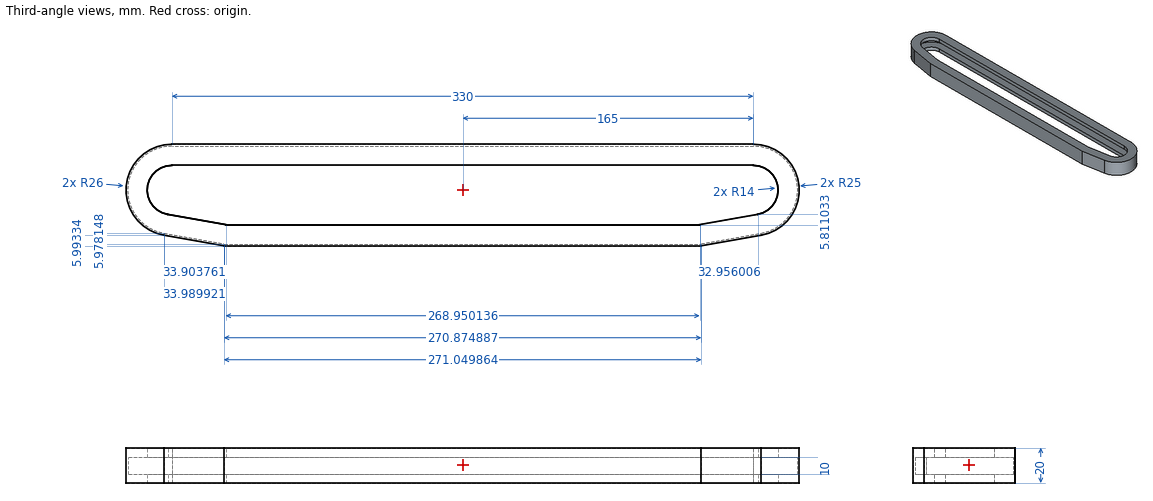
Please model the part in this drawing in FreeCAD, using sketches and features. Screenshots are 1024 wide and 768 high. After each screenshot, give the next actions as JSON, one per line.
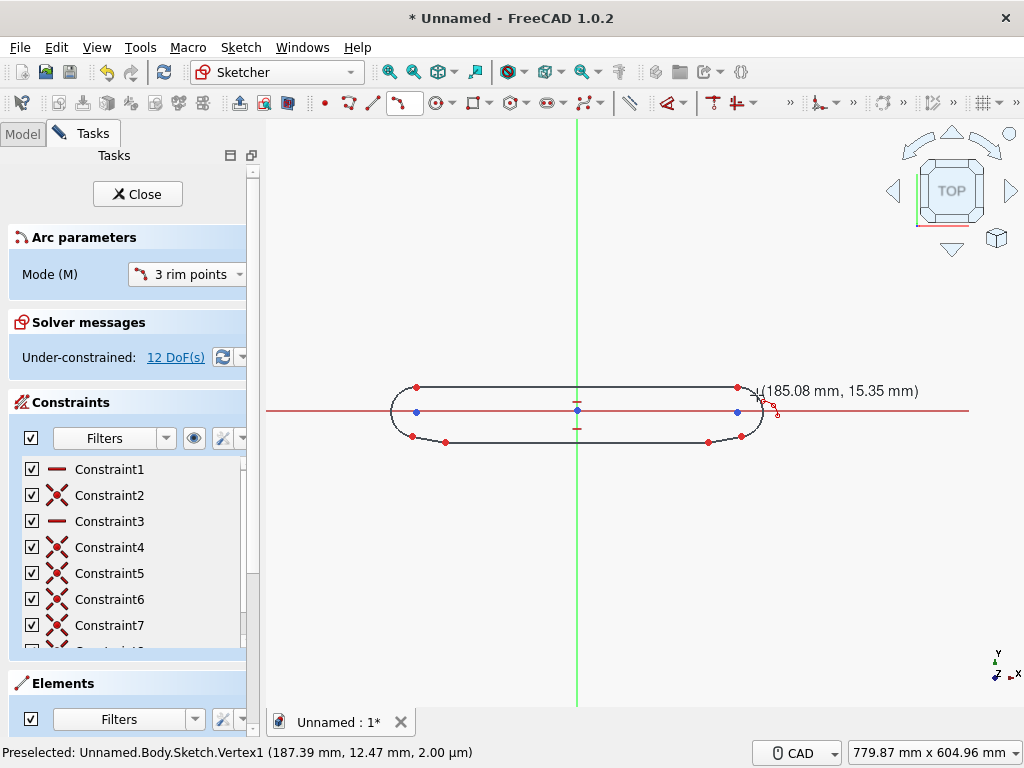
{"action": "left_click", "coordinate": [374, 104]}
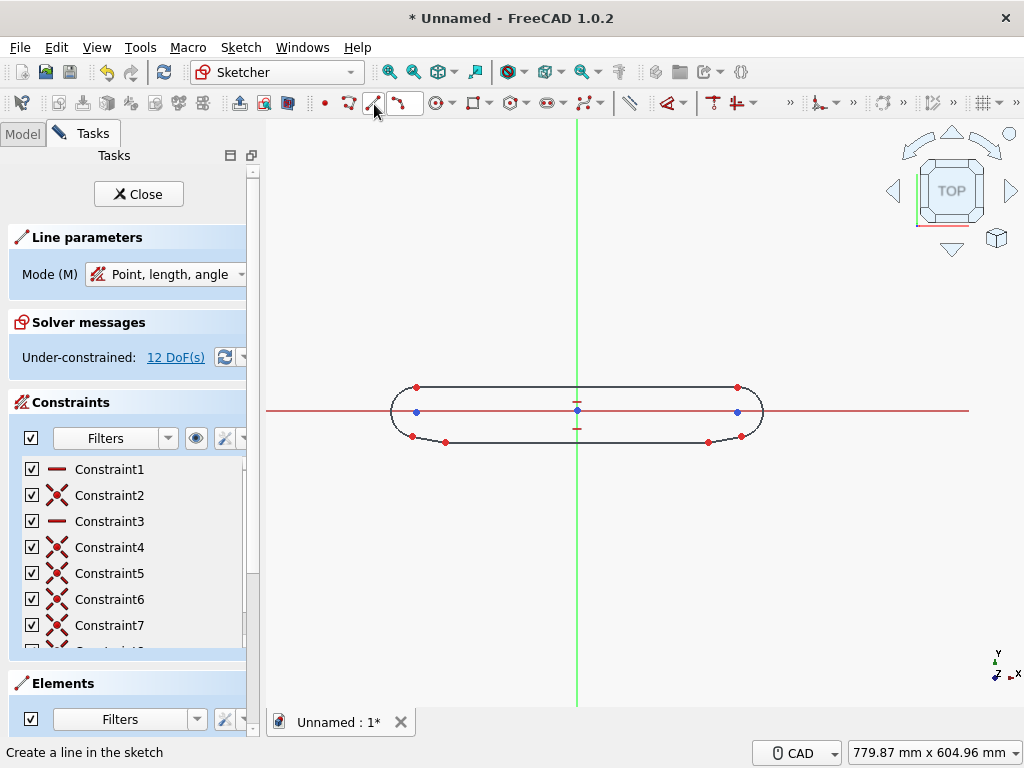
{"action": "scroll", "coordinate": [417, 397], "scroll_direction": "up", "scroll_amount": 2}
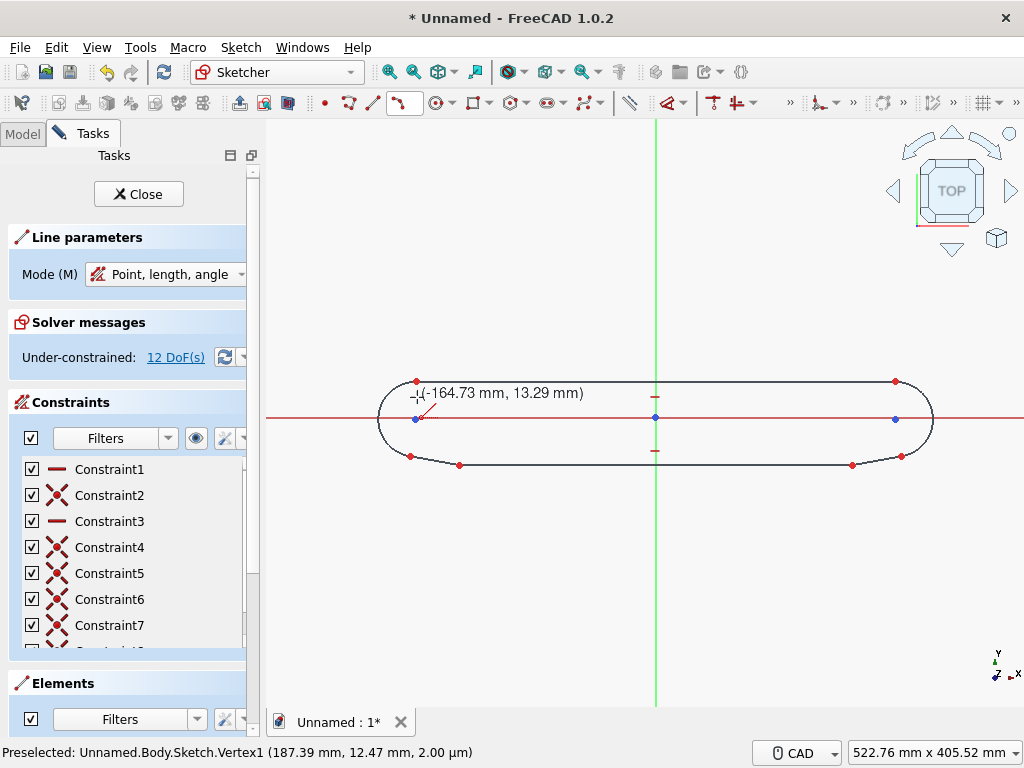
{"action": "left_click", "coordinate": [417, 397]}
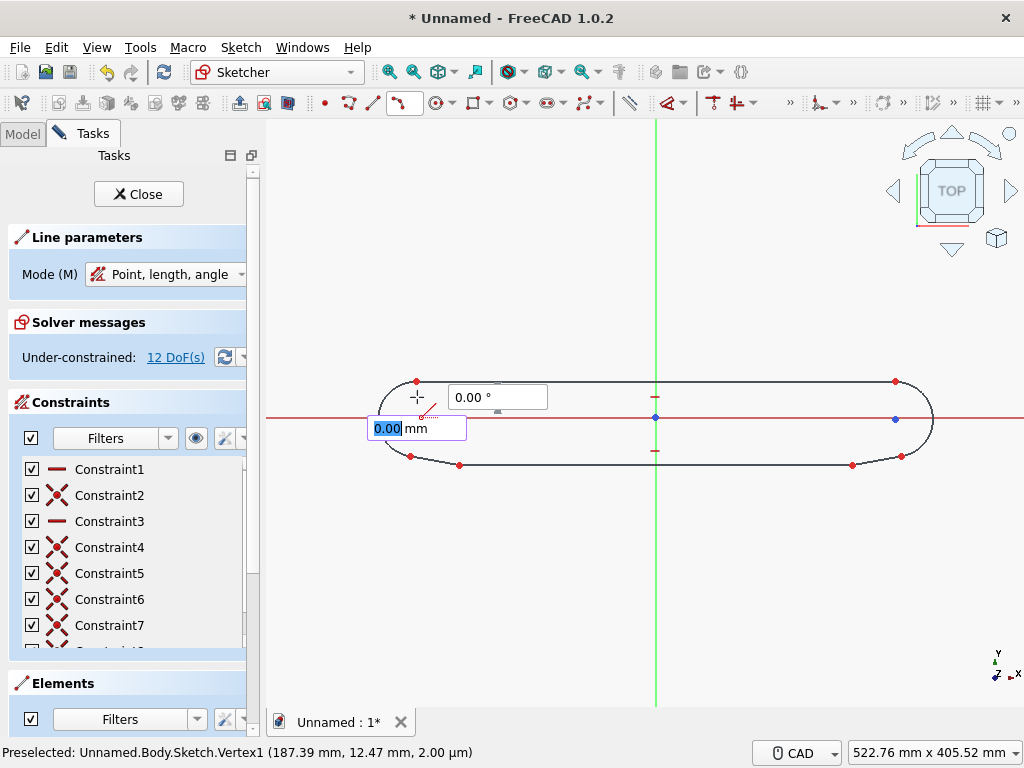
{"action": "scroll", "coordinate": [415, 396], "scroll_direction": "down", "scroll_amount": 2}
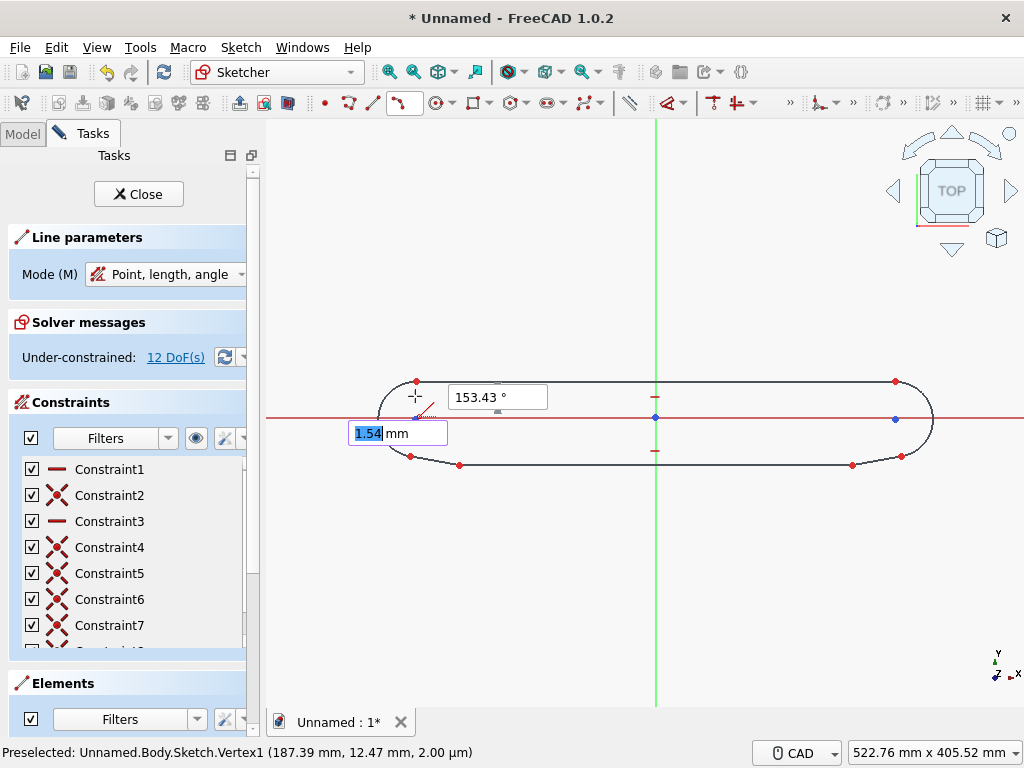
{"action": "scroll", "coordinate": [737, 397], "scroll_direction": "up", "scroll_amount": 2}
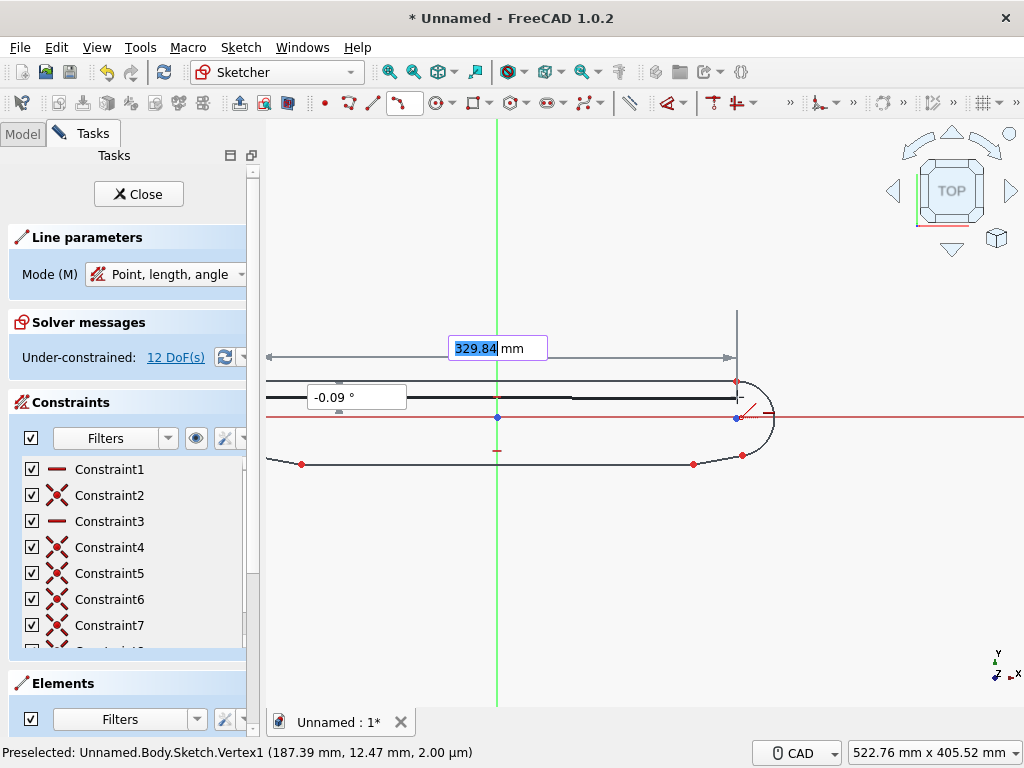
{"action": "left_click", "coordinate": [736, 397]}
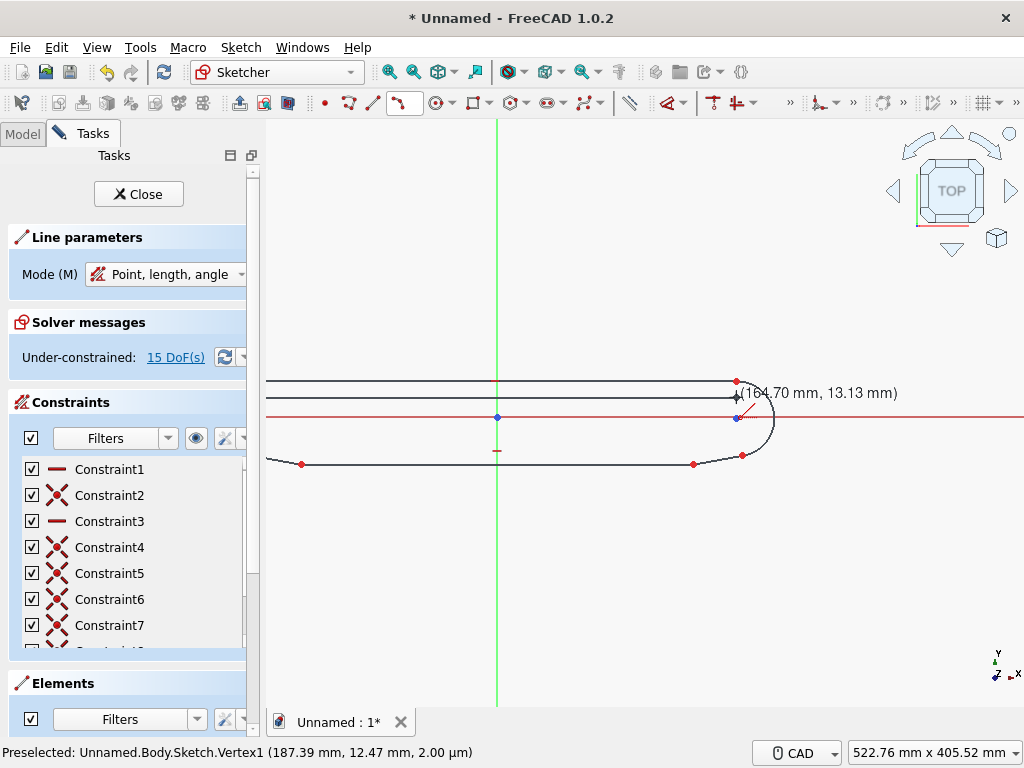
{"action": "left_click", "coordinate": [350, 104]}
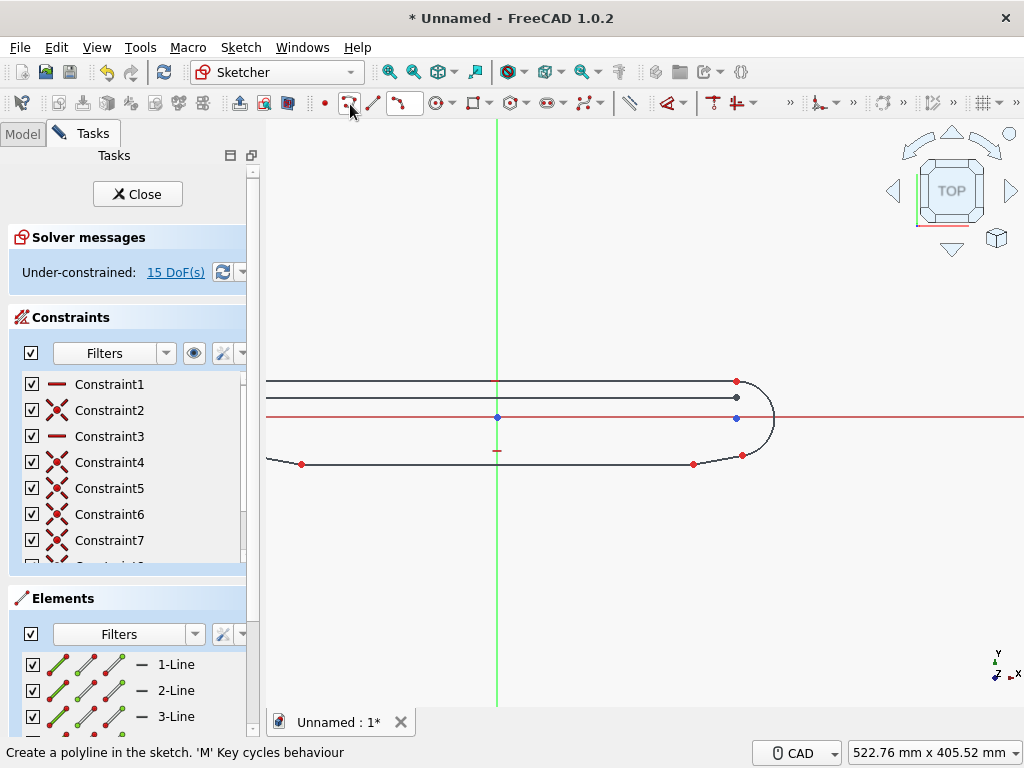
{"action": "left_click", "coordinate": [740, 437]}
{"action": "left_click", "coordinate": [692, 445]}
{"action": "left_click", "coordinate": [302, 445]}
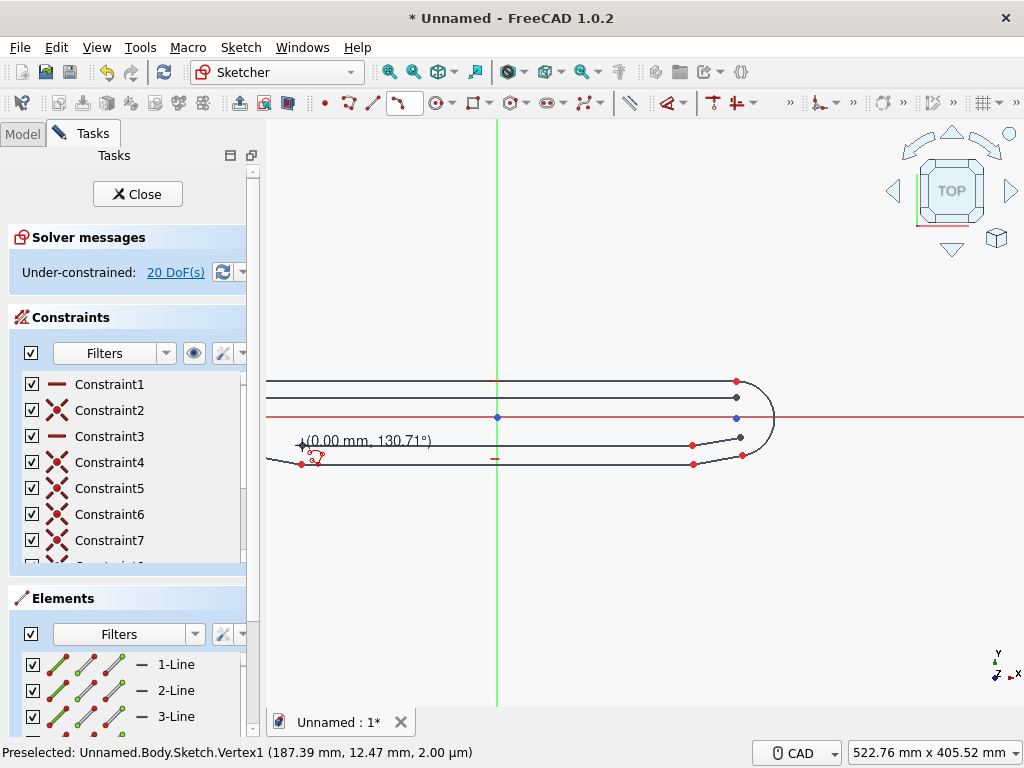
{"action": "scroll", "coordinate": [738, 397], "scroll_direction": "down", "scroll_amount": 2}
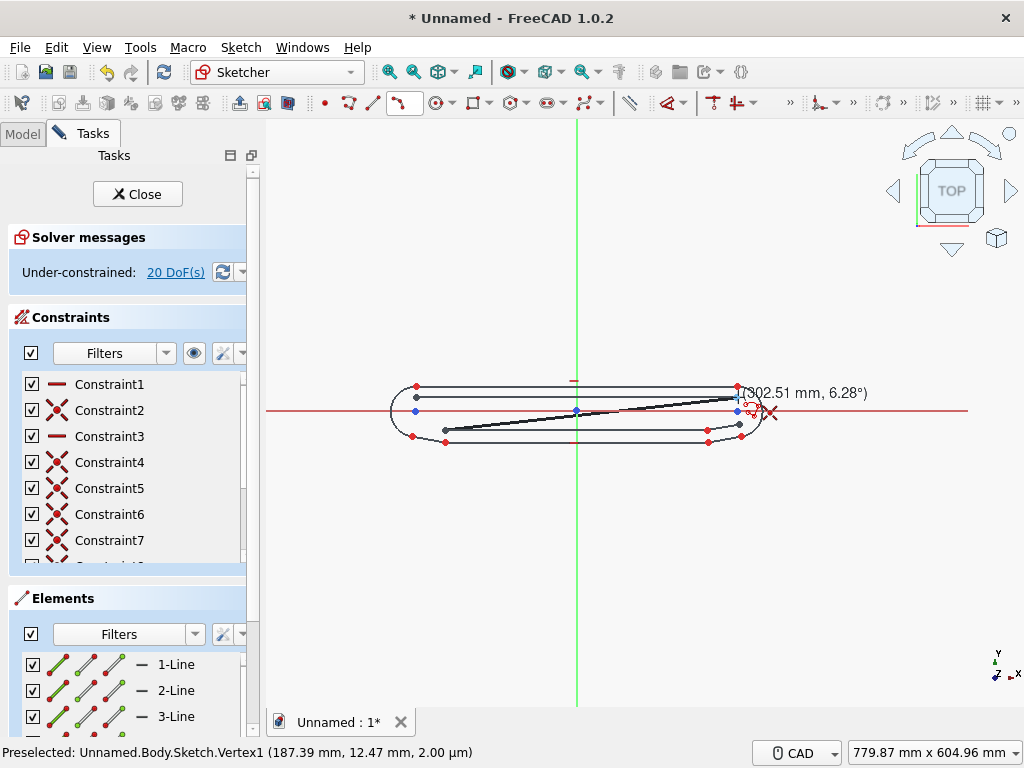
{"action": "scroll", "coordinate": [414, 424], "scroll_direction": "up", "scroll_amount": 2}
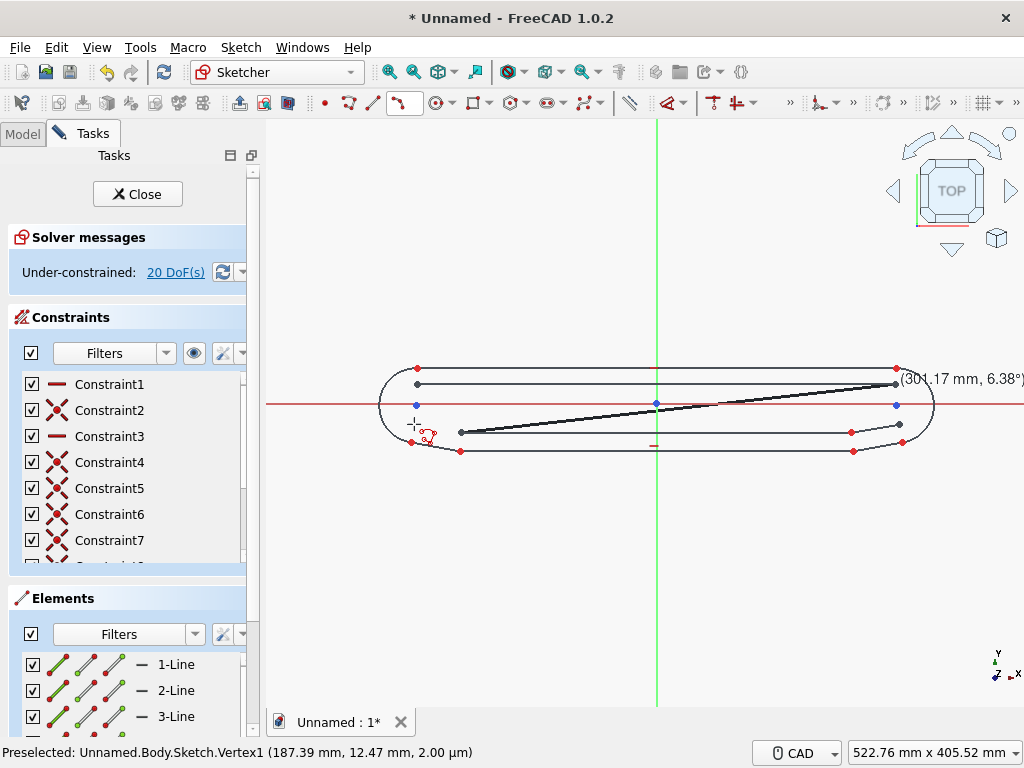
{"action": "left_click", "coordinate": [414, 424]}
{"action": "right_click", "coordinate": [414, 424]}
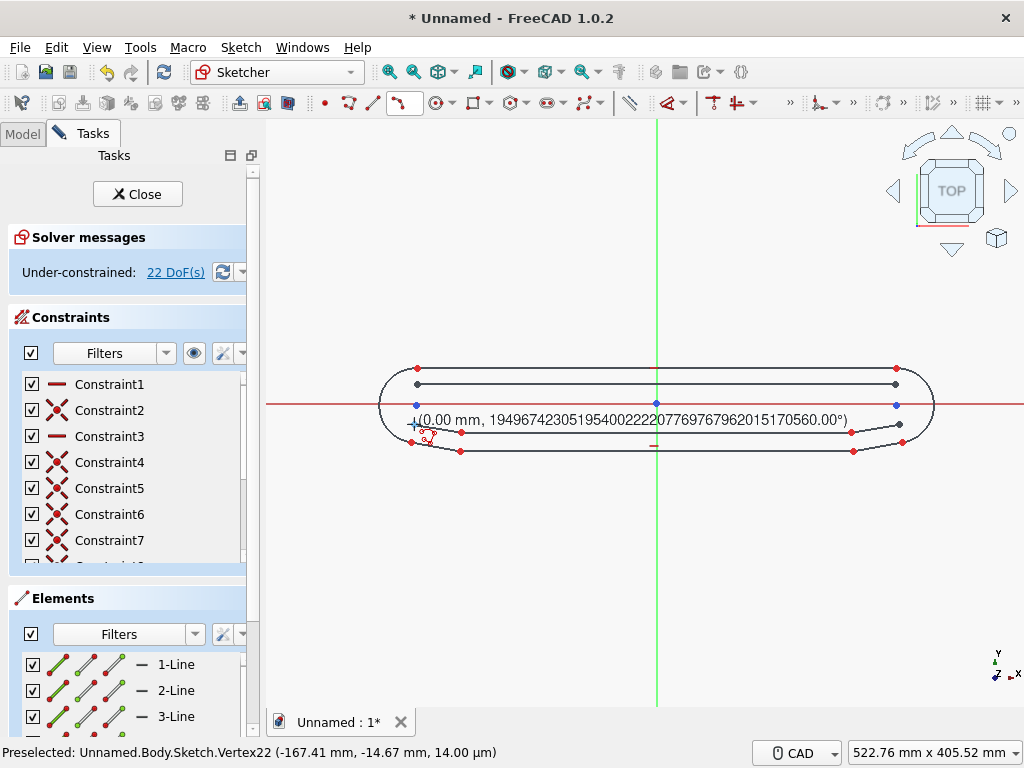
{"action": "left_click", "coordinate": [398, 104]}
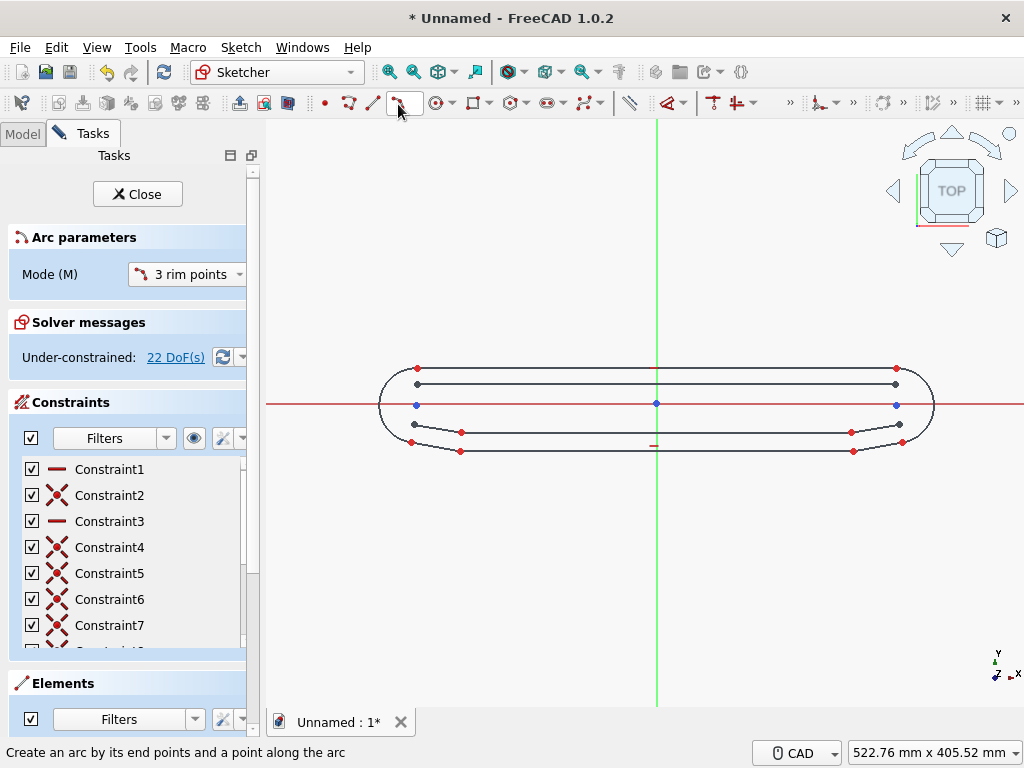
{"action": "scroll", "coordinate": [413, 424], "scroll_direction": "down", "scroll_amount": 2}